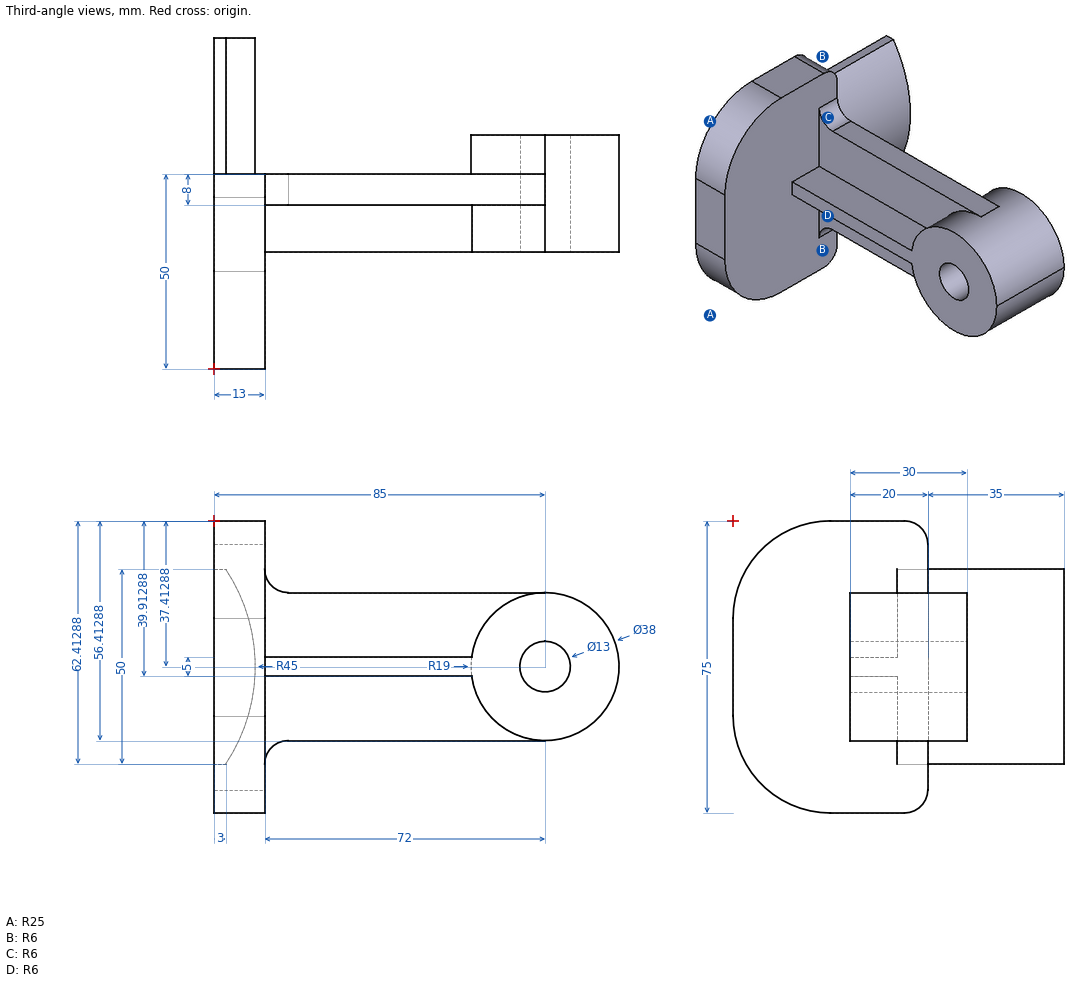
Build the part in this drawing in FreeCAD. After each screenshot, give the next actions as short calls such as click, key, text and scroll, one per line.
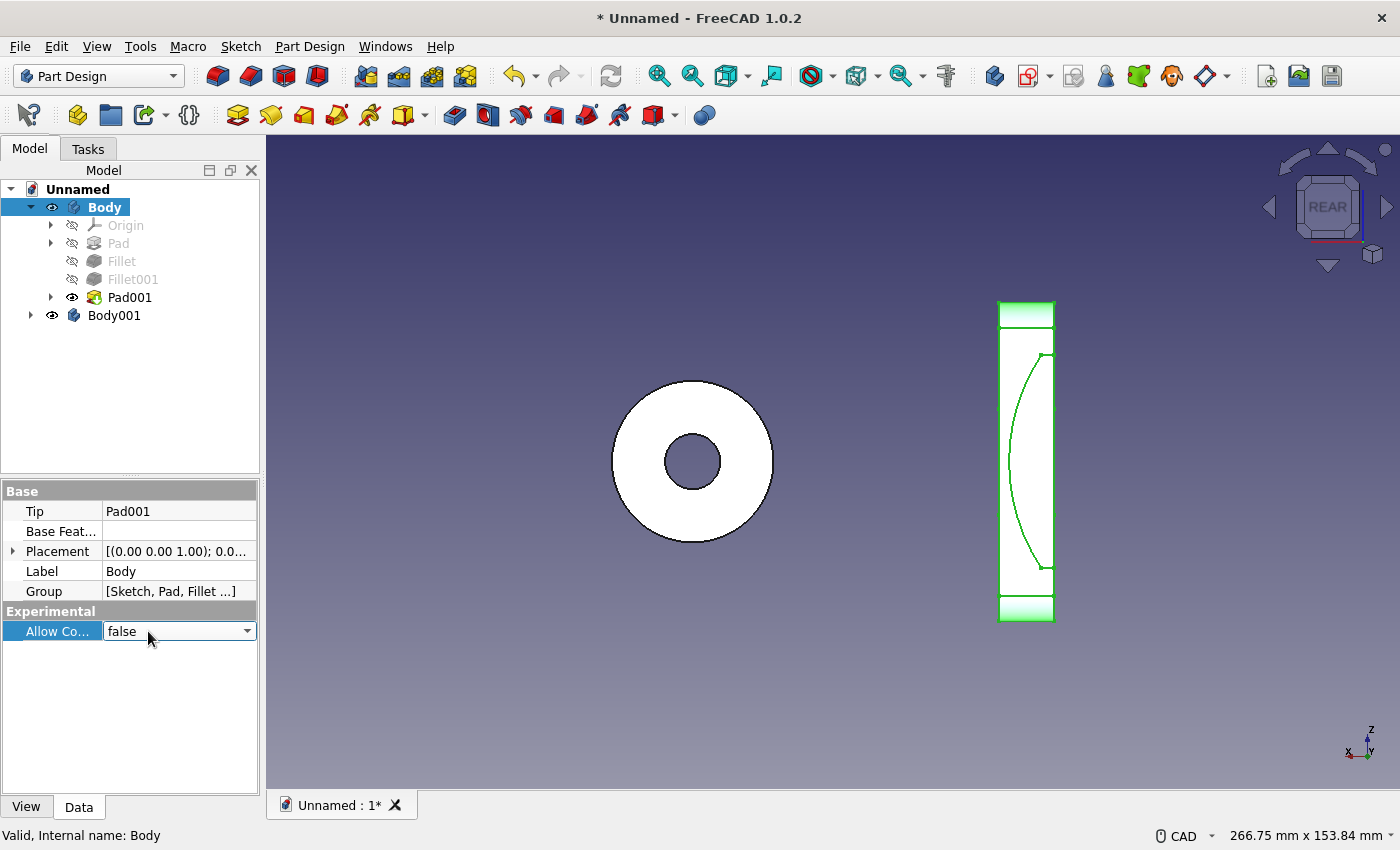
click(148, 631)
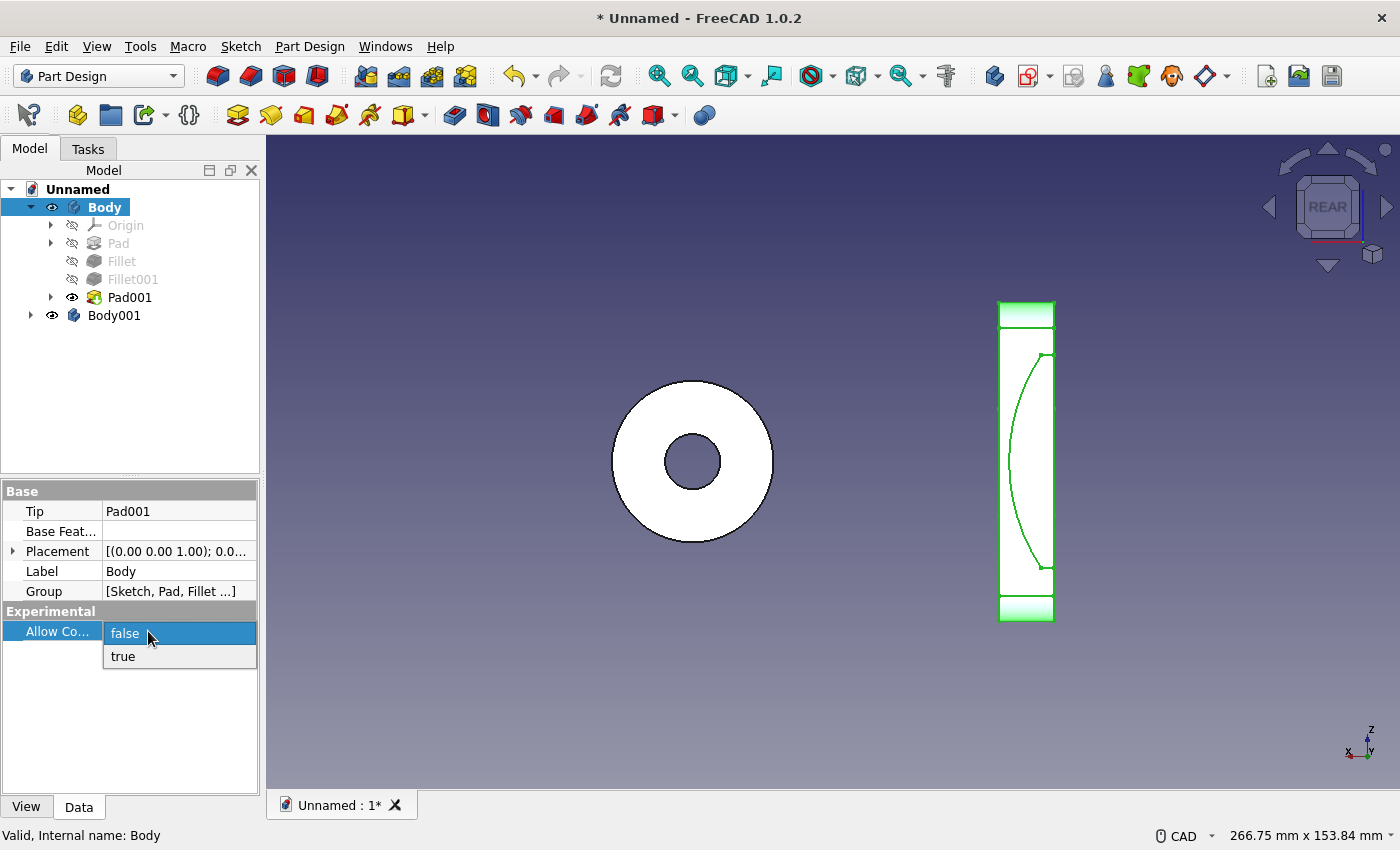
click(178, 656)
key(Return)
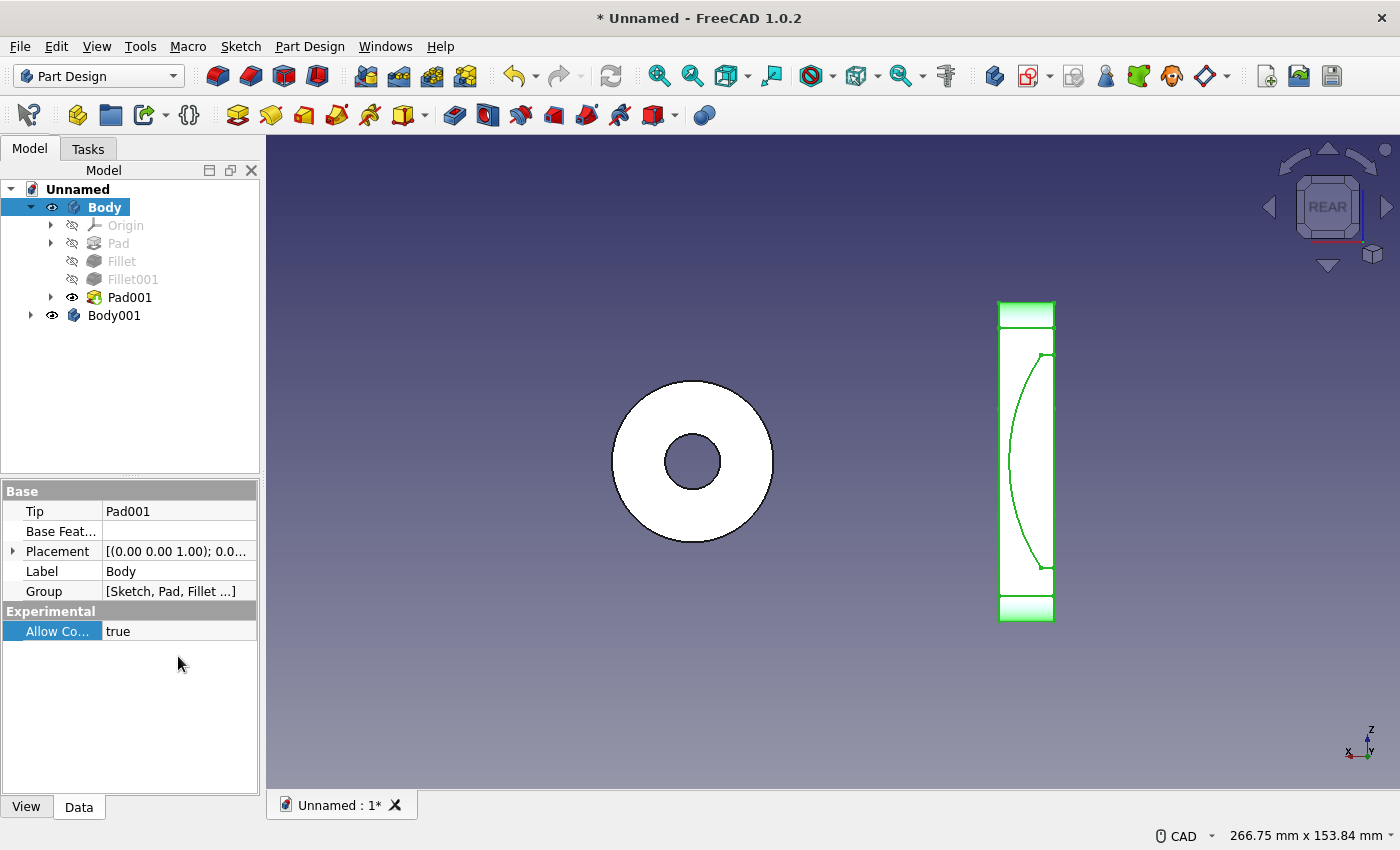
click(97, 315)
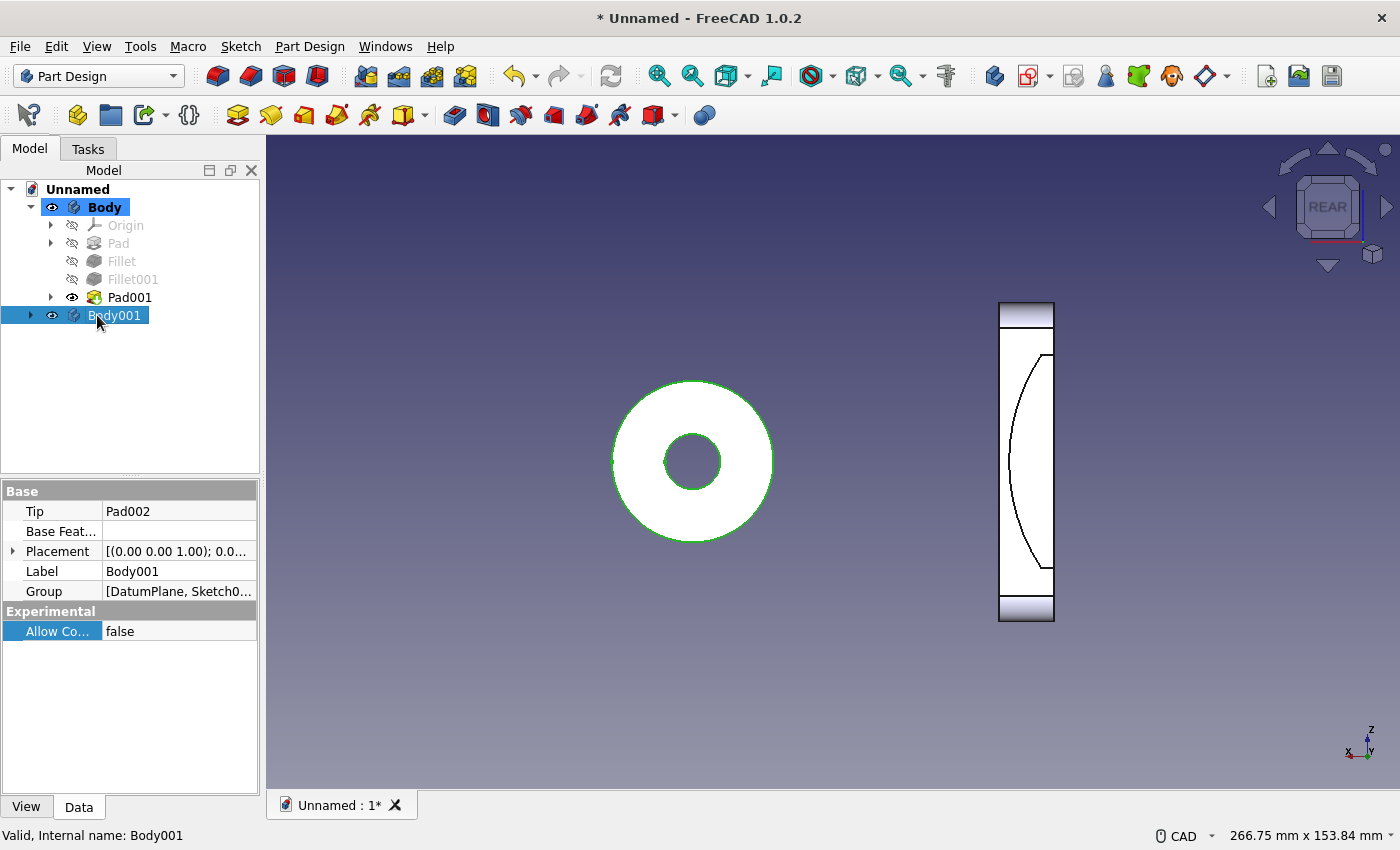
click(705, 116)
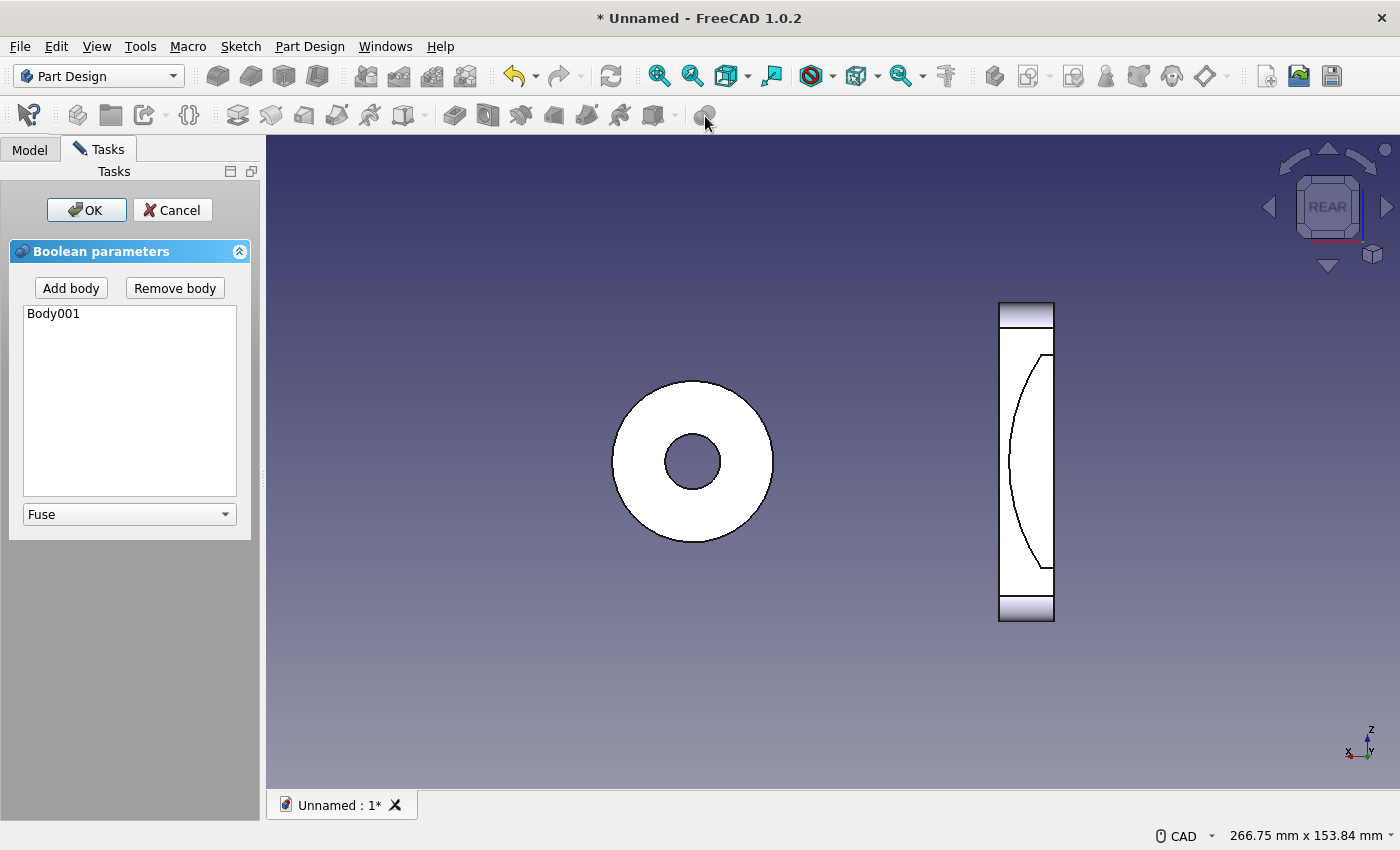
click(87, 210)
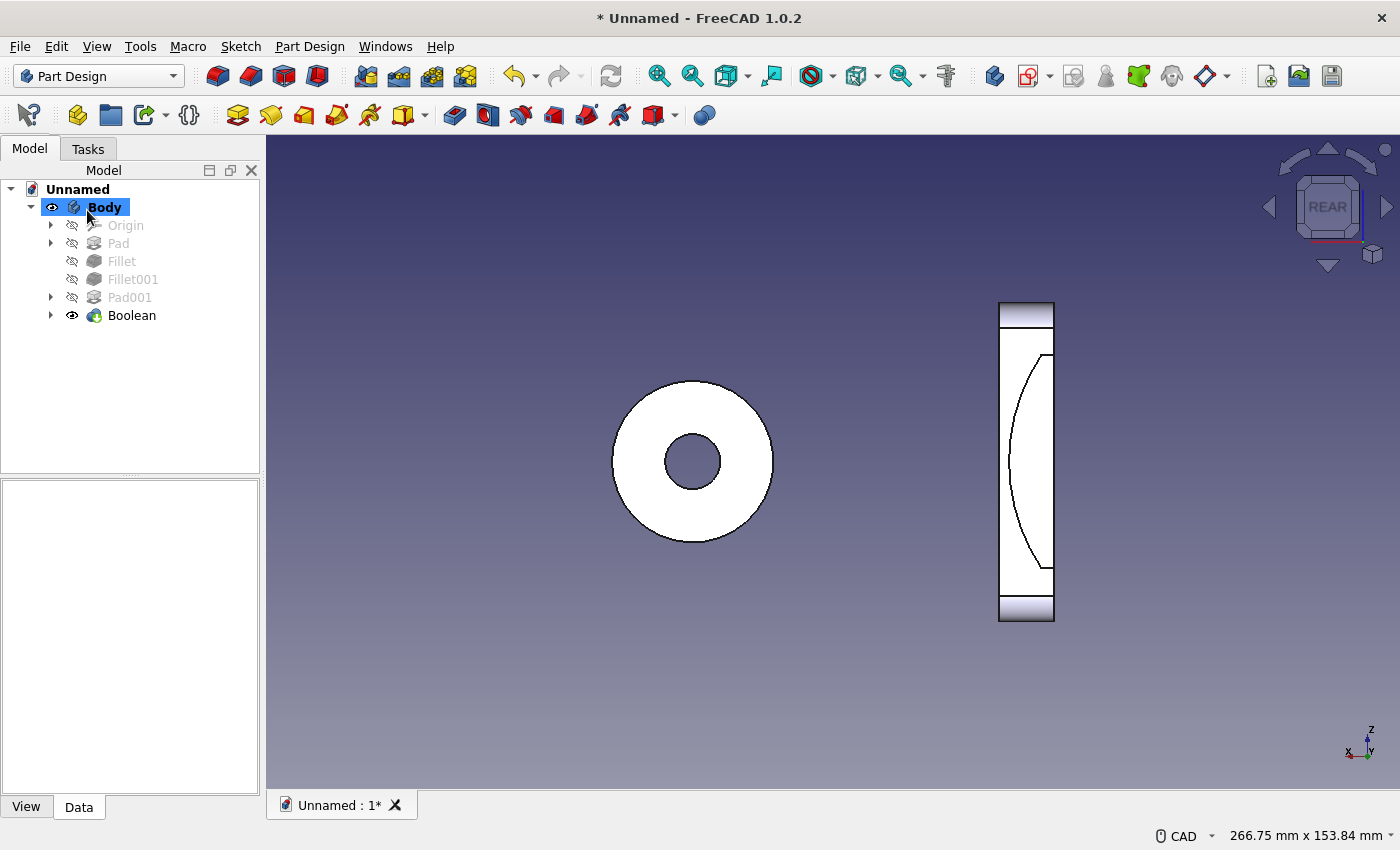
click(1019, 346)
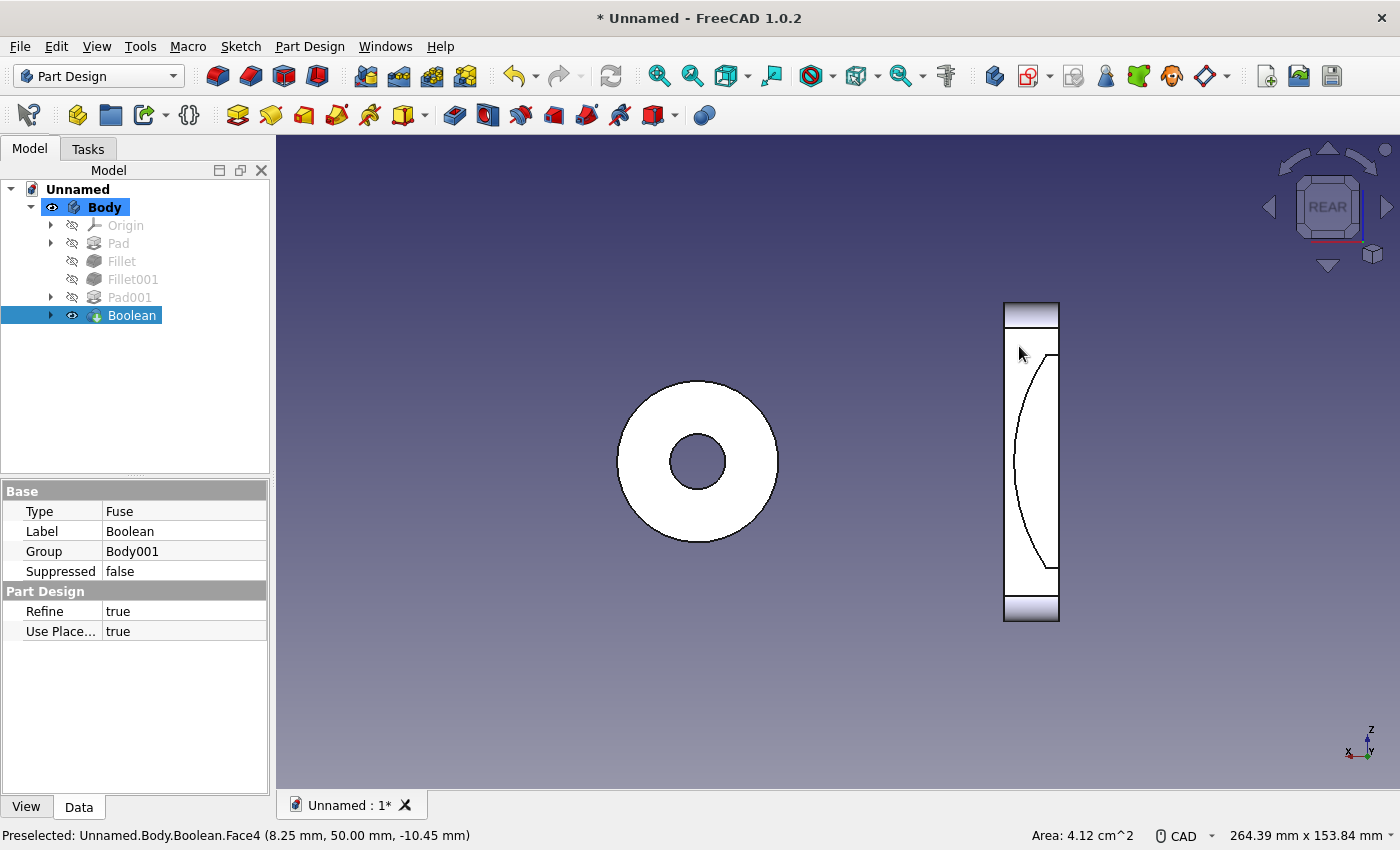
click(1028, 76)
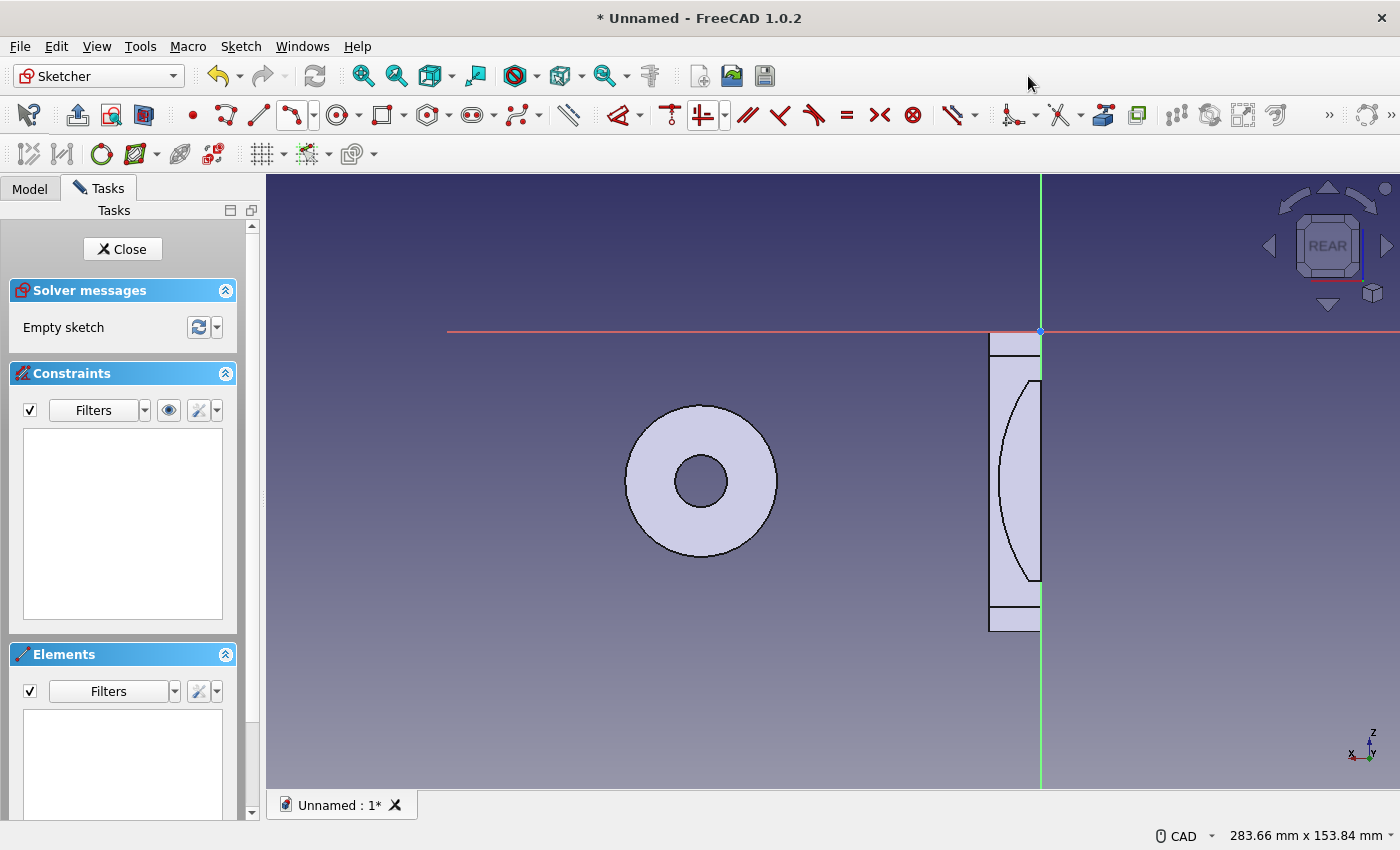
click(144, 116)